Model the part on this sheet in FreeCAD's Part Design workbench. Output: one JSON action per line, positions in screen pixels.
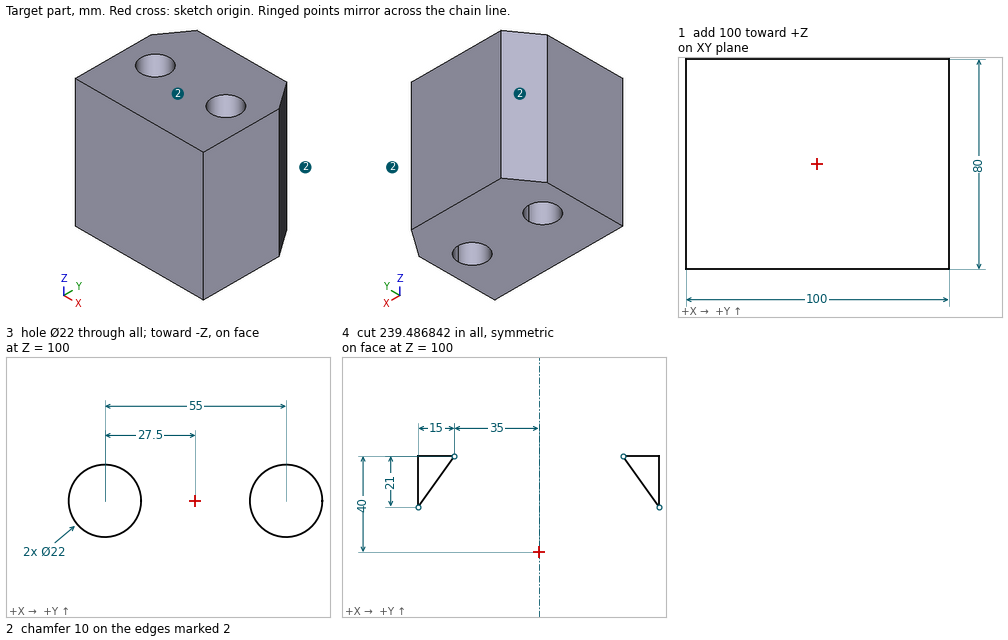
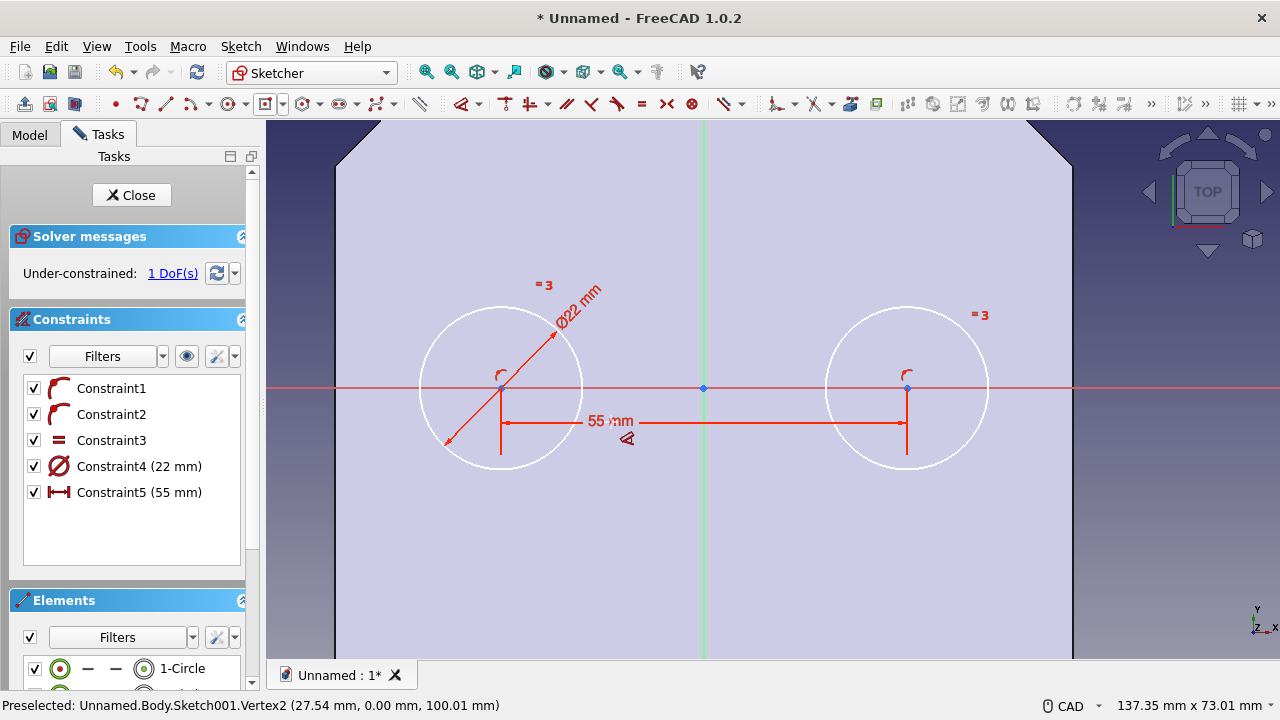
{"action": "left_click", "coordinate": [501, 388]}
{"action": "left_click", "coordinate": [531, 422]}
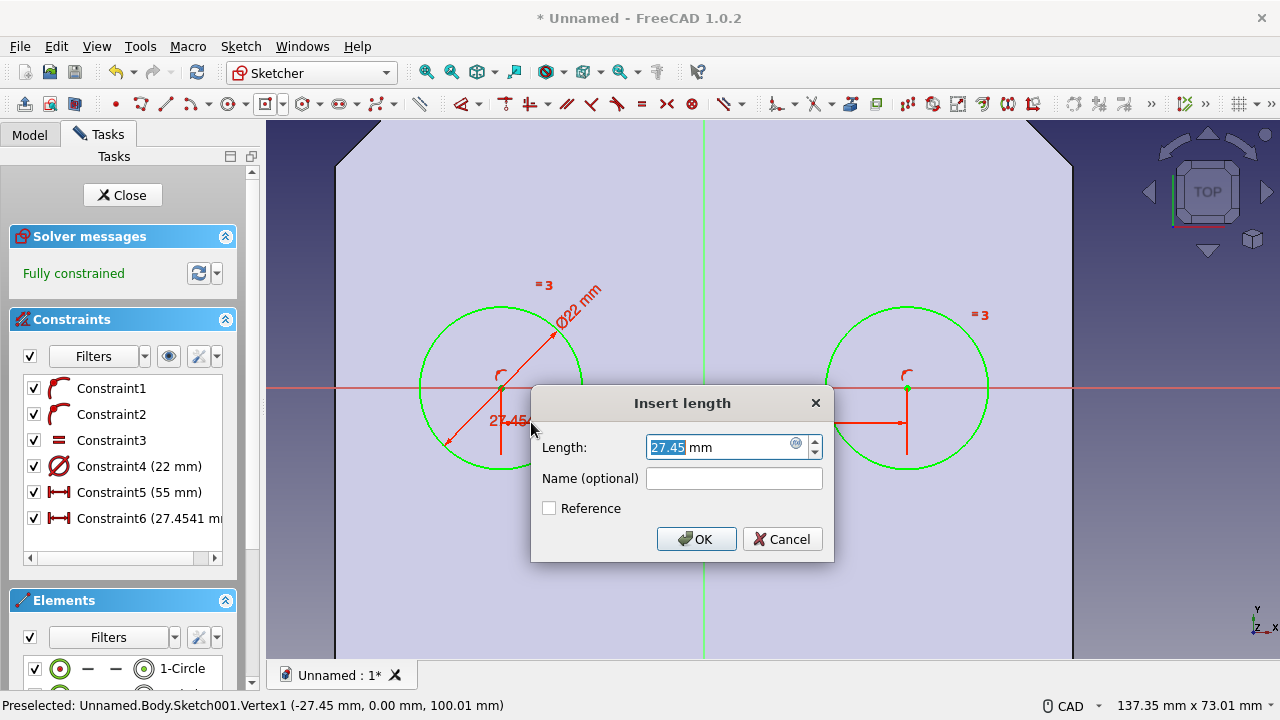
{"action": "type", "text": "27.5"}
{"action": "key", "text": "Return"}
{"action": "key", "text": "Escape"}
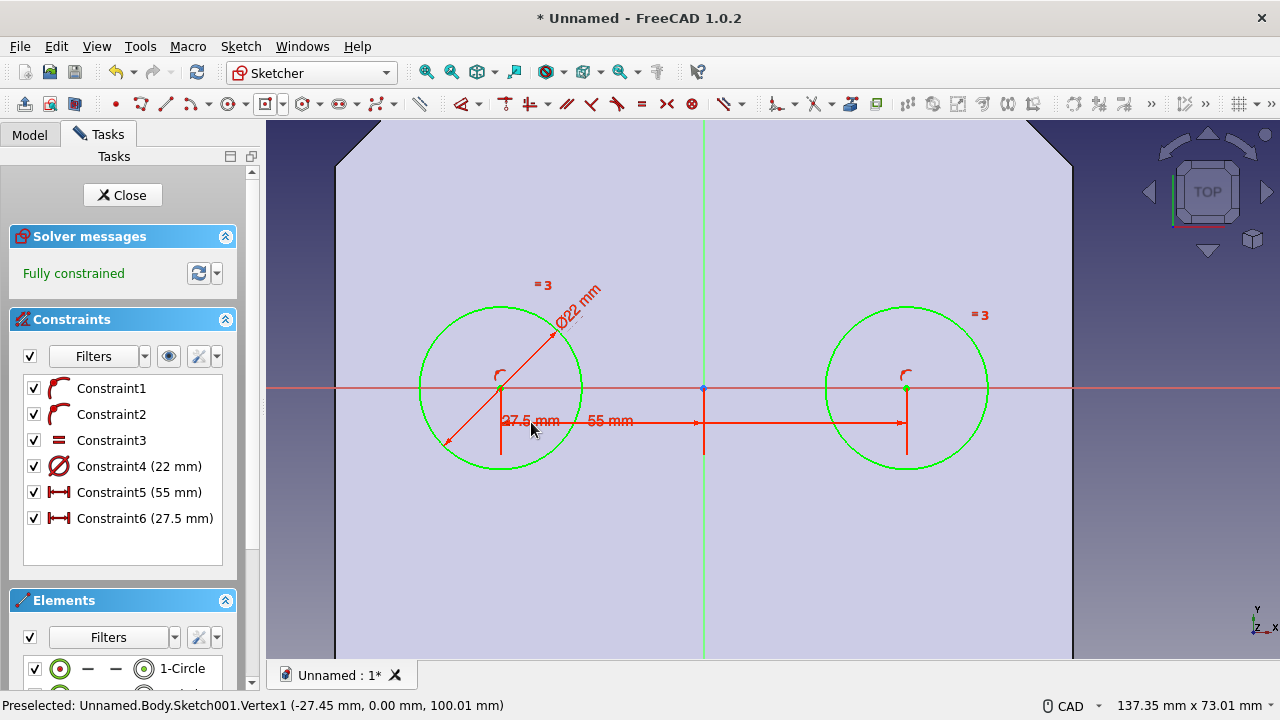
{"action": "left_click", "coordinate": [123, 195]}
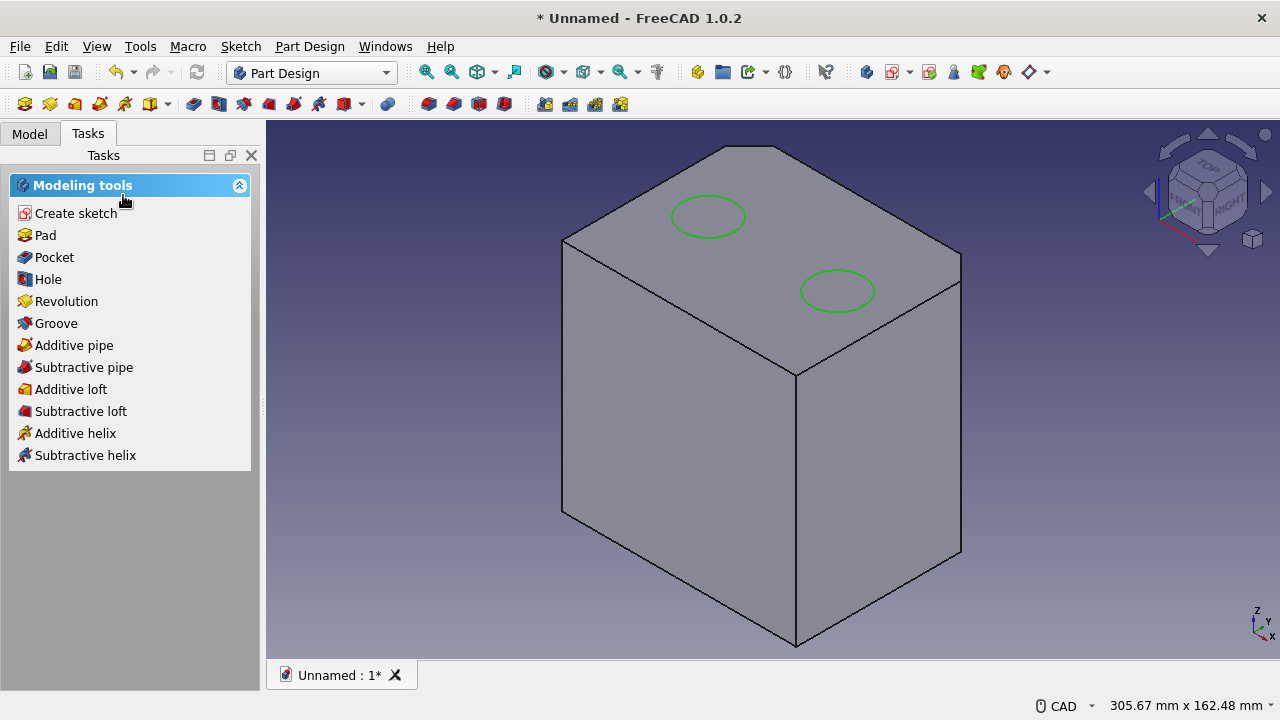
{"action": "left_click", "coordinate": [219, 104]}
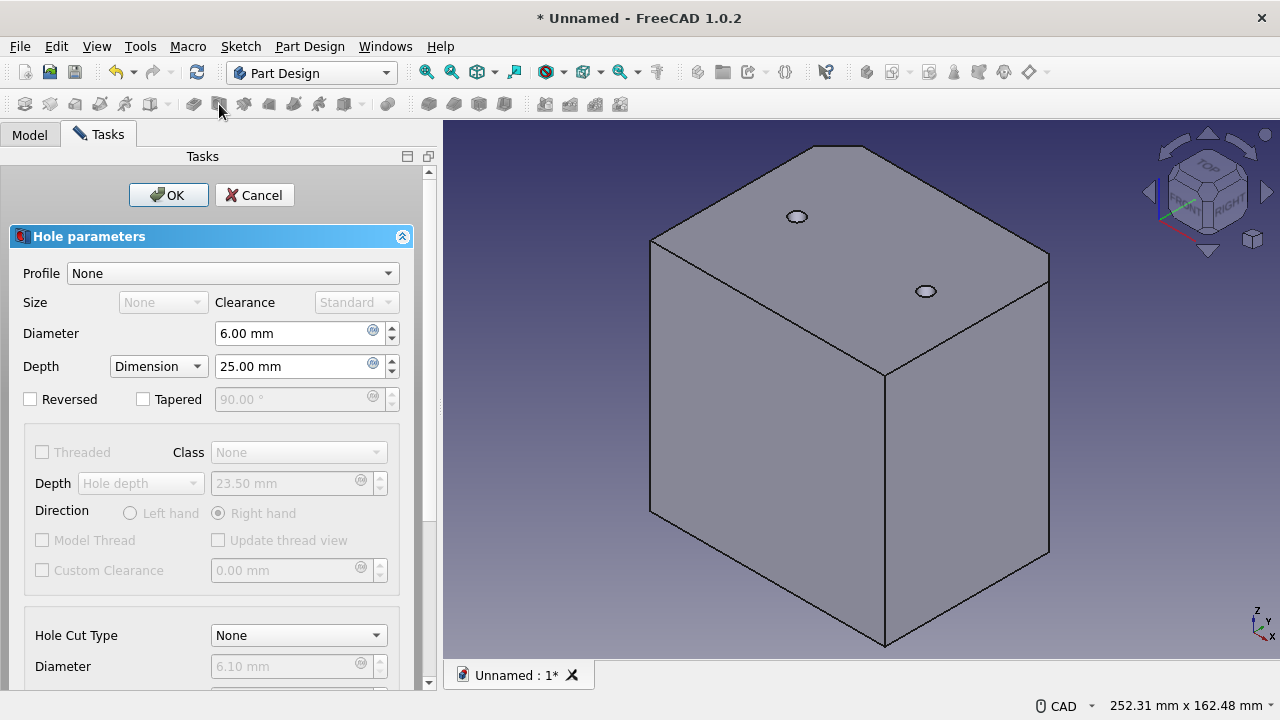
{"action": "triple_click", "coordinate": [300, 334]}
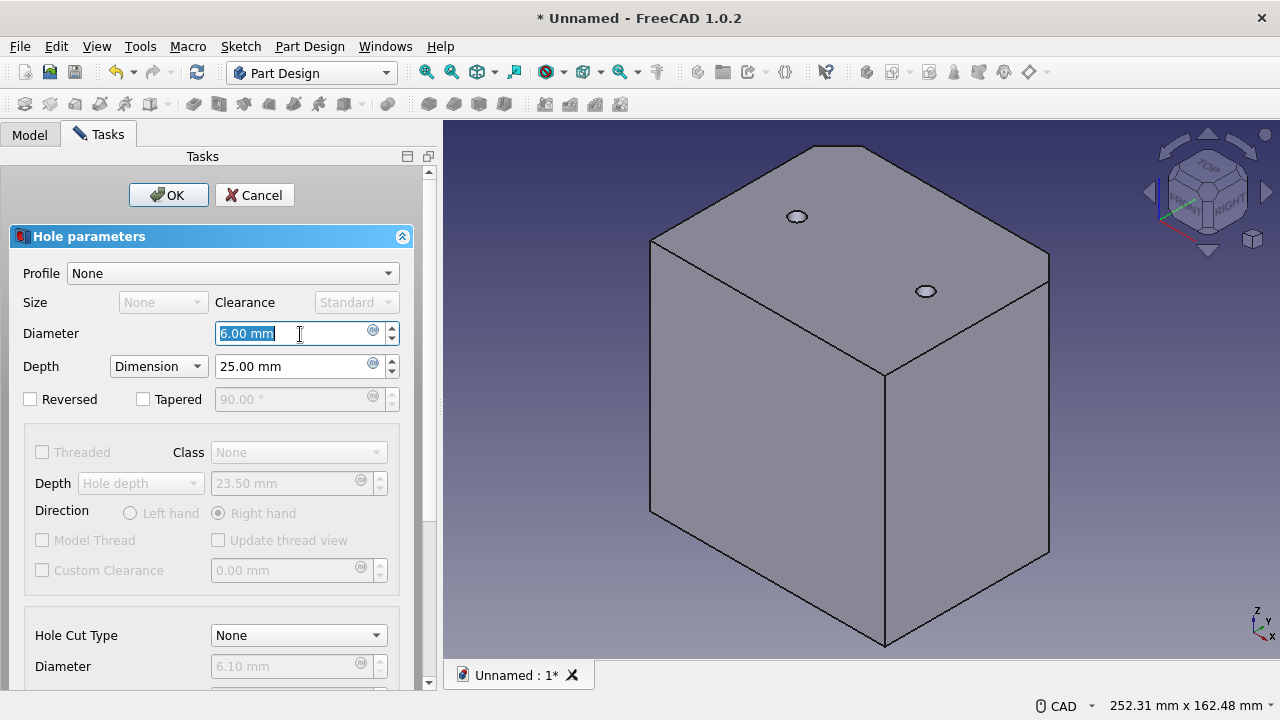
{"action": "type", "text": "22"}
{"action": "key", "text": "Tab"}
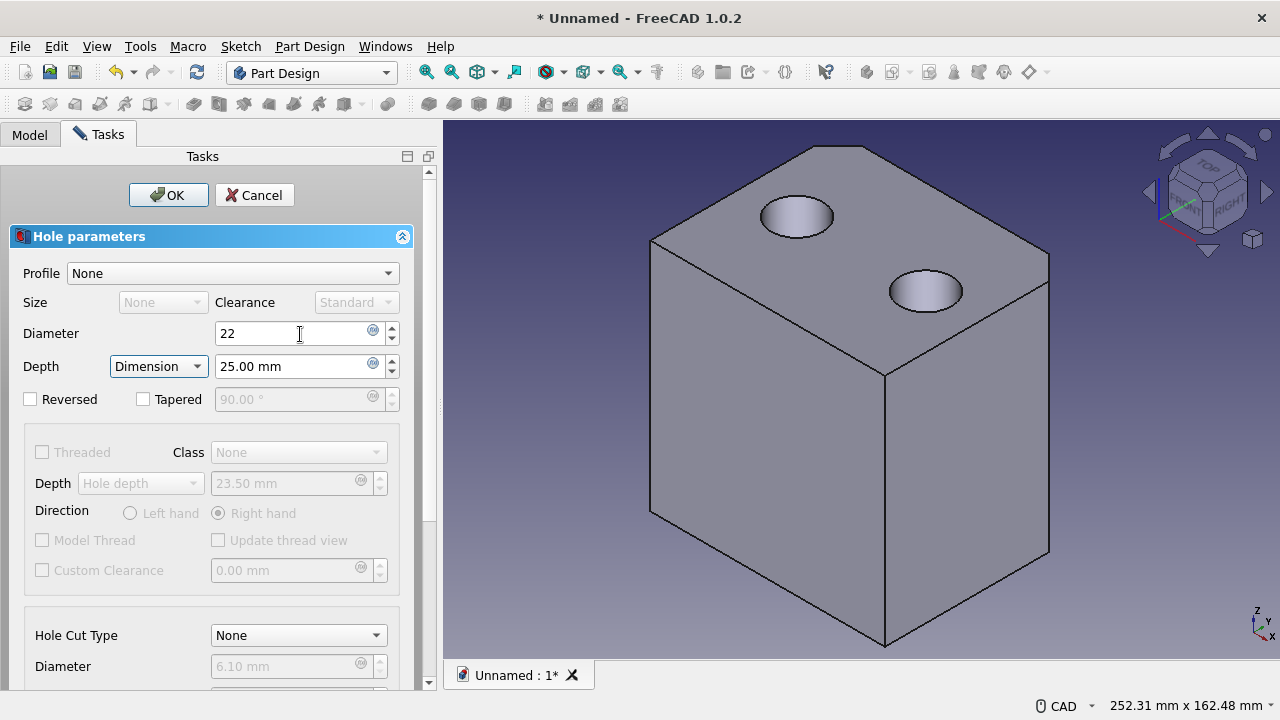
{"action": "left_click", "coordinate": [160, 366]}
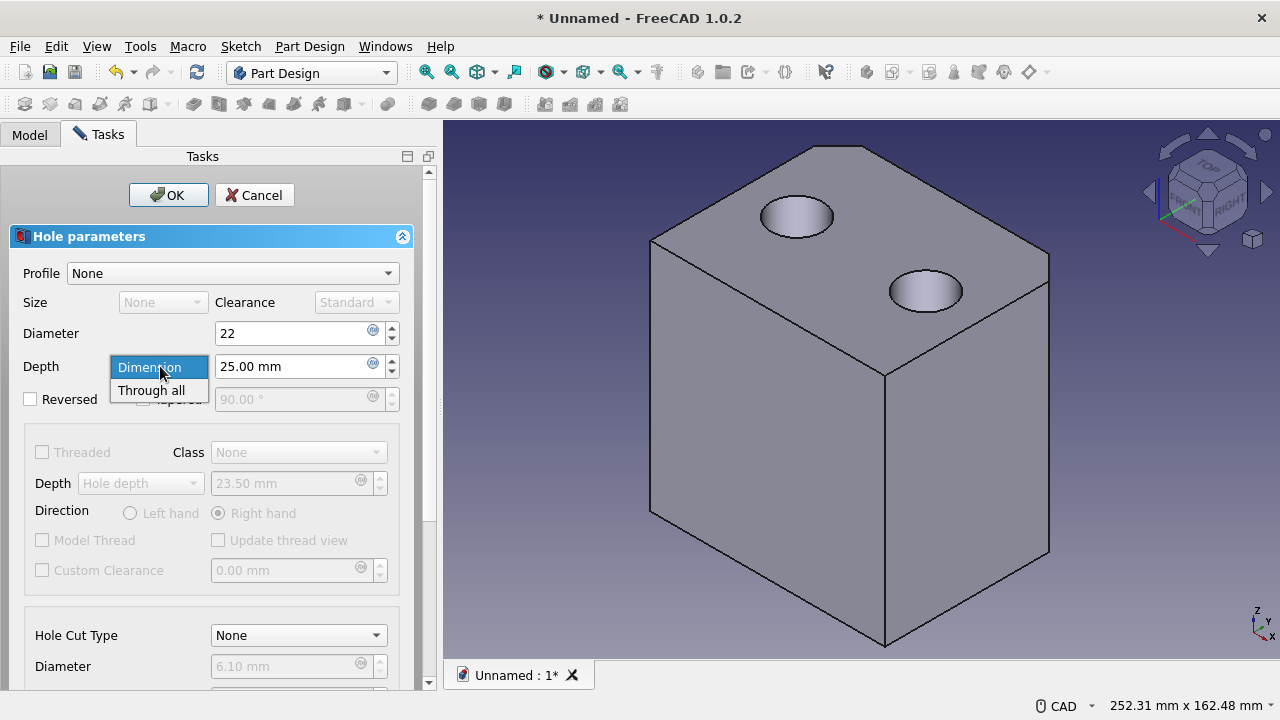
{"action": "left_click", "coordinate": [158, 390]}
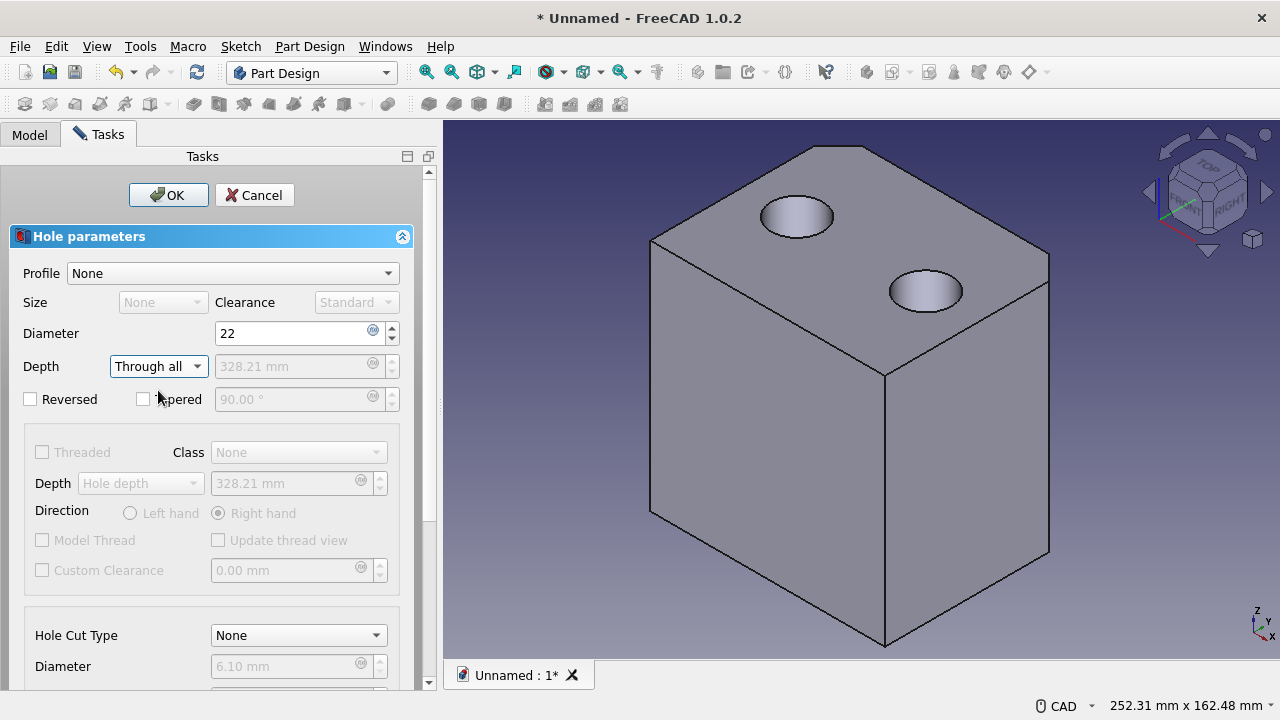
{"action": "left_click", "coordinate": [169, 195]}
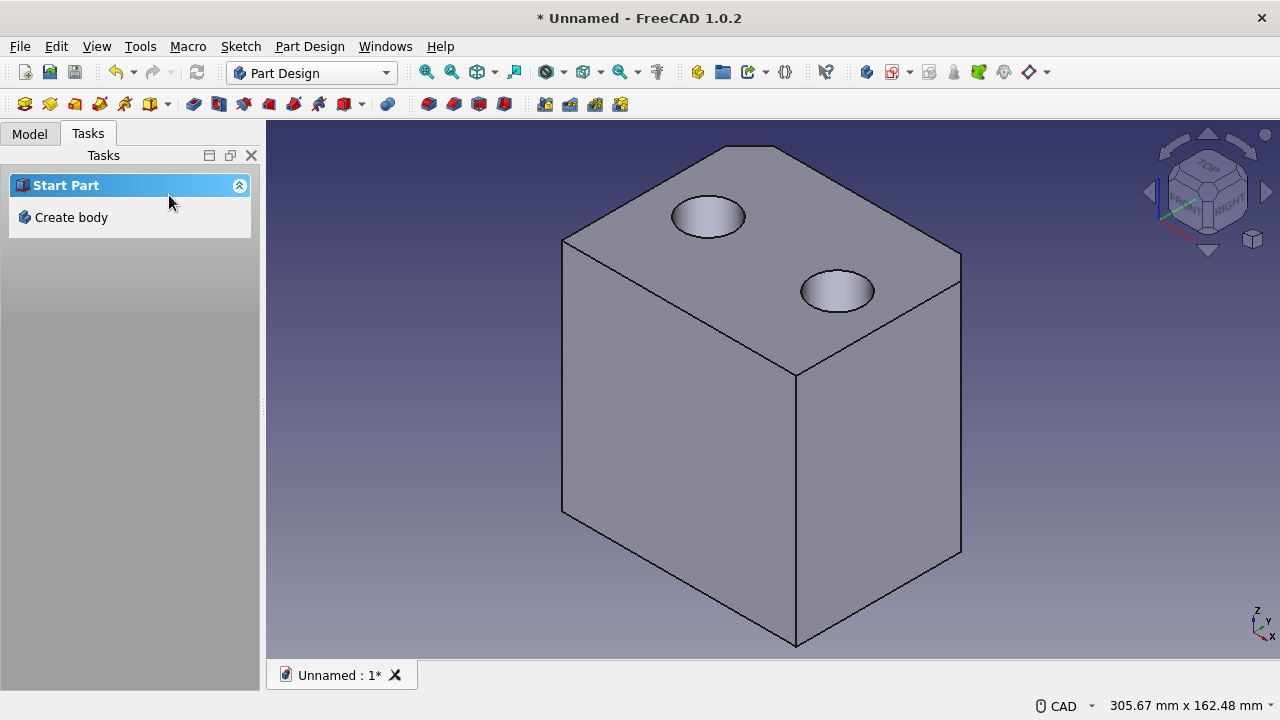
{"action": "left_click", "coordinate": [800, 238]}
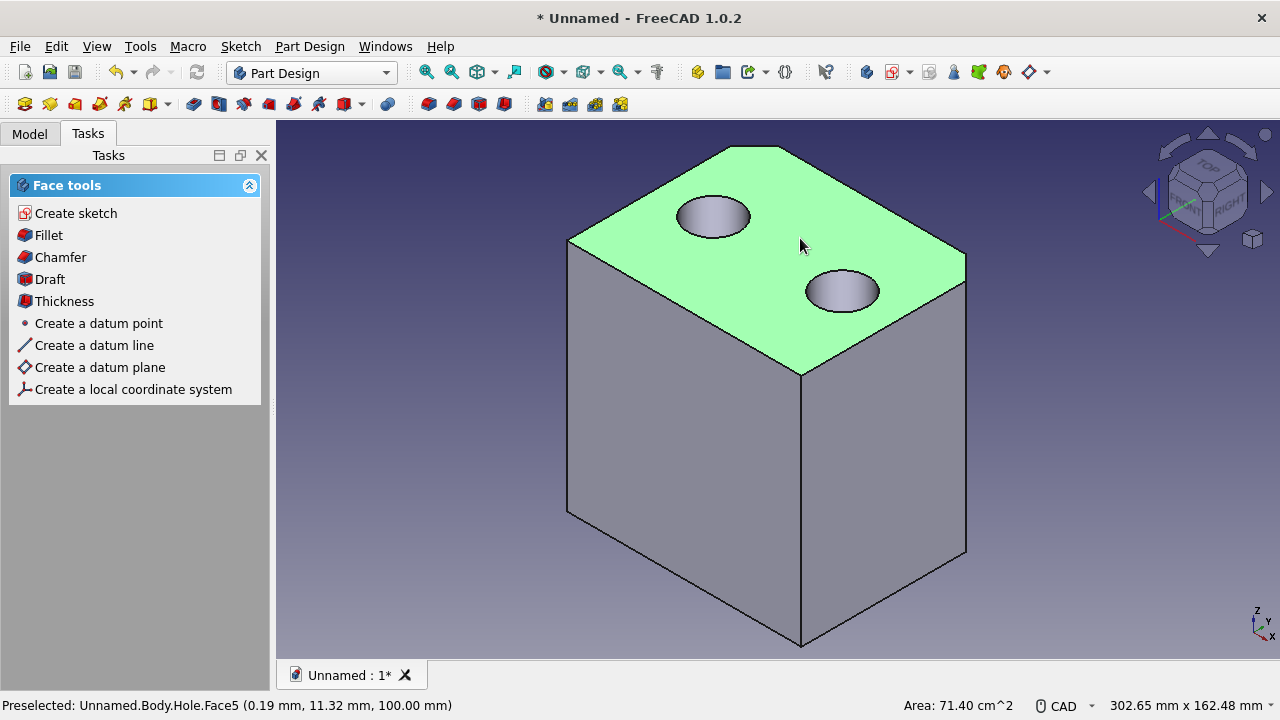
{"action": "left_click", "coordinate": [892, 72]}